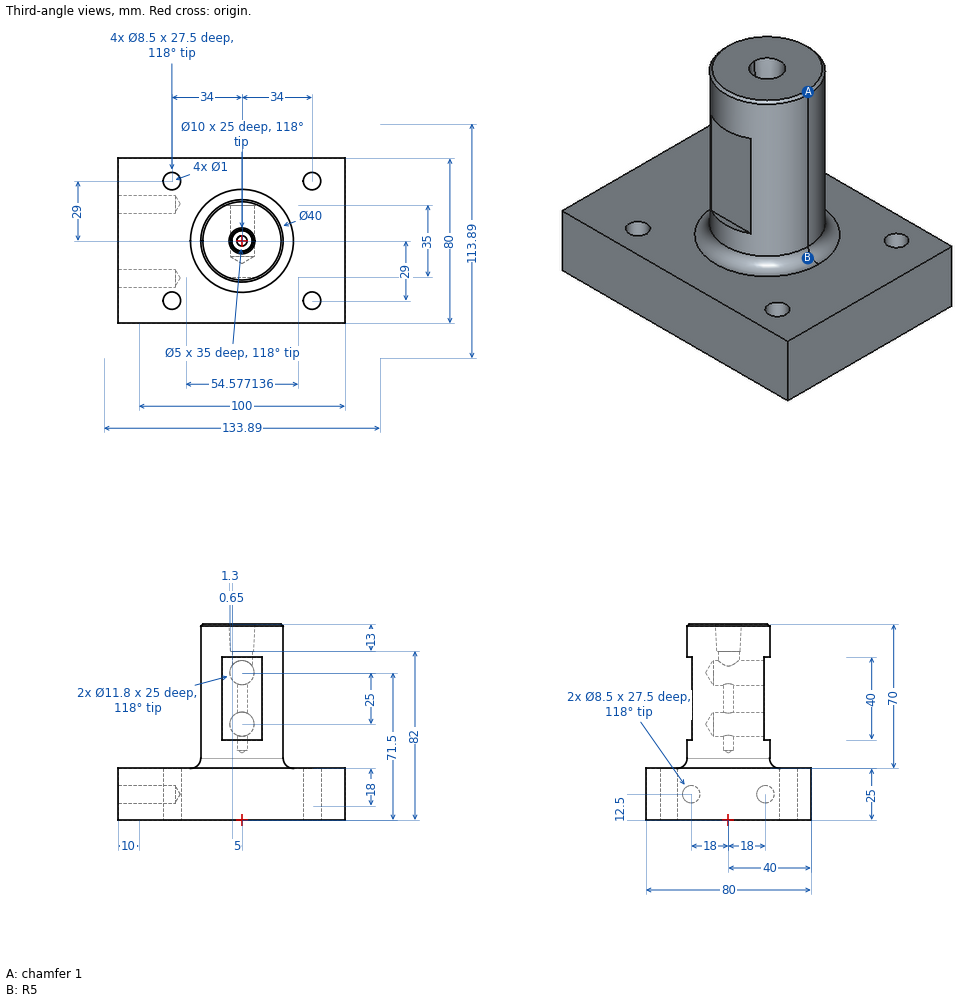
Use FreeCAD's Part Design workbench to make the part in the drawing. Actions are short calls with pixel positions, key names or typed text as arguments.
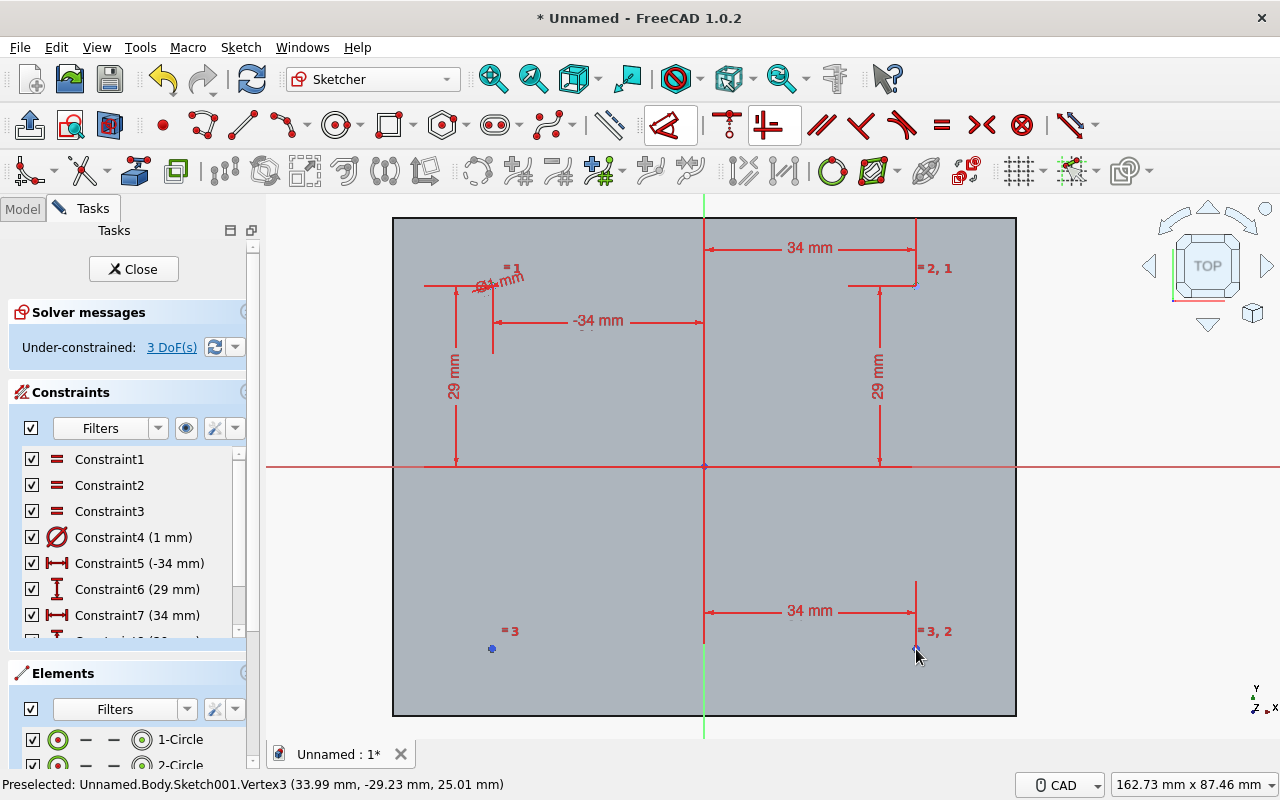
click(916, 649)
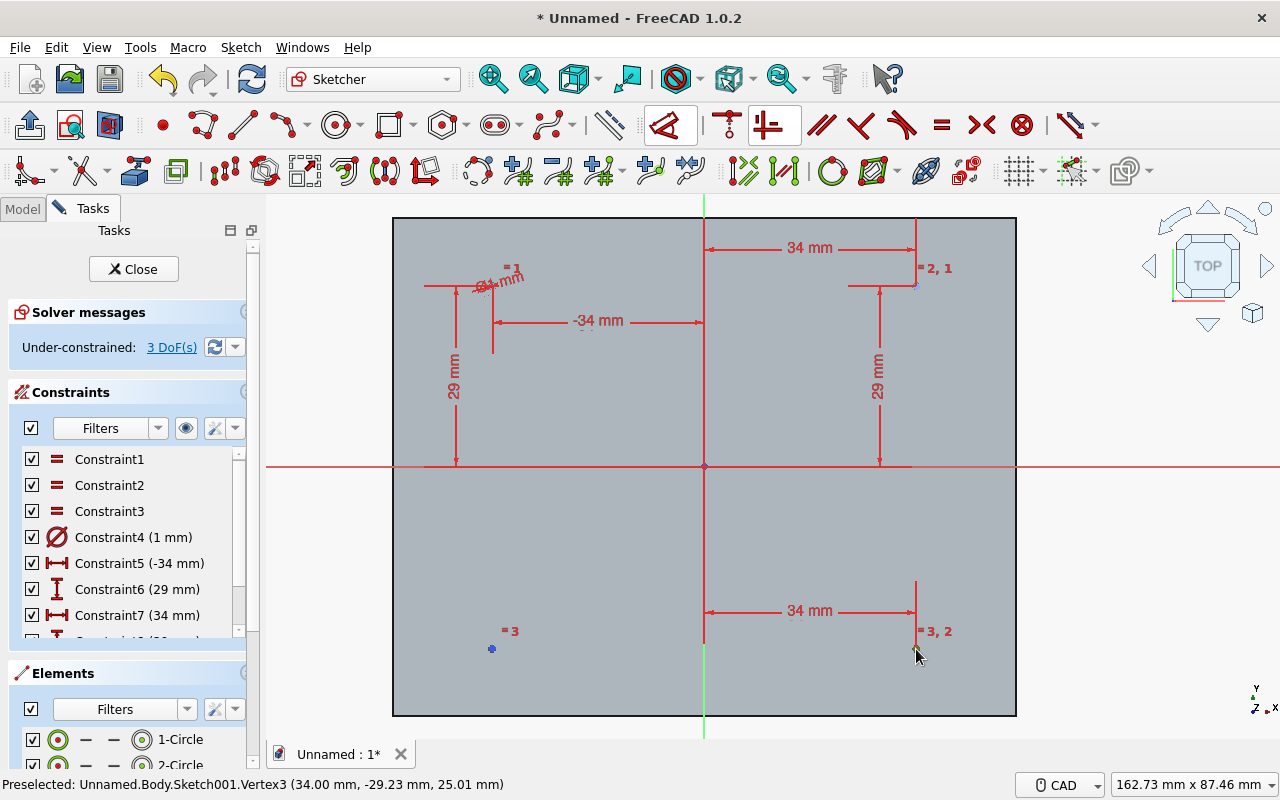
key(i)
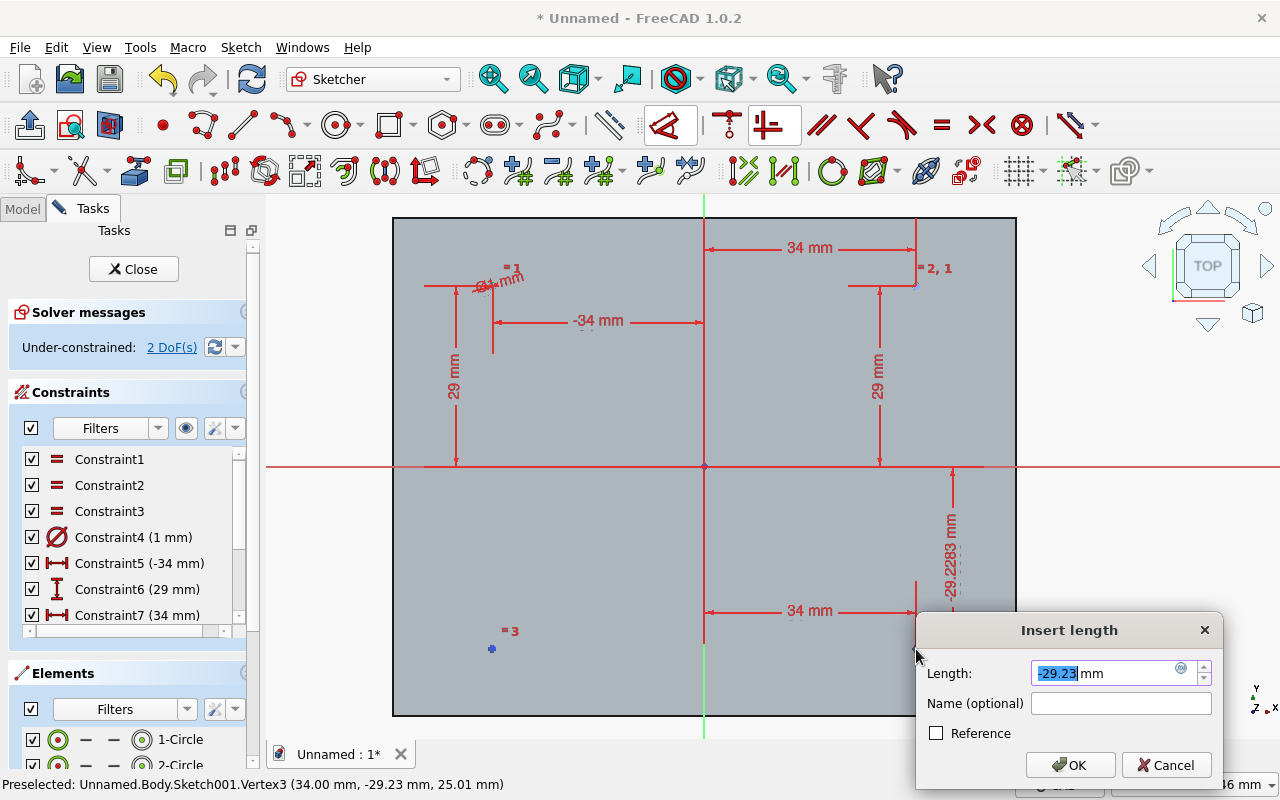
text(-29)
key(Return)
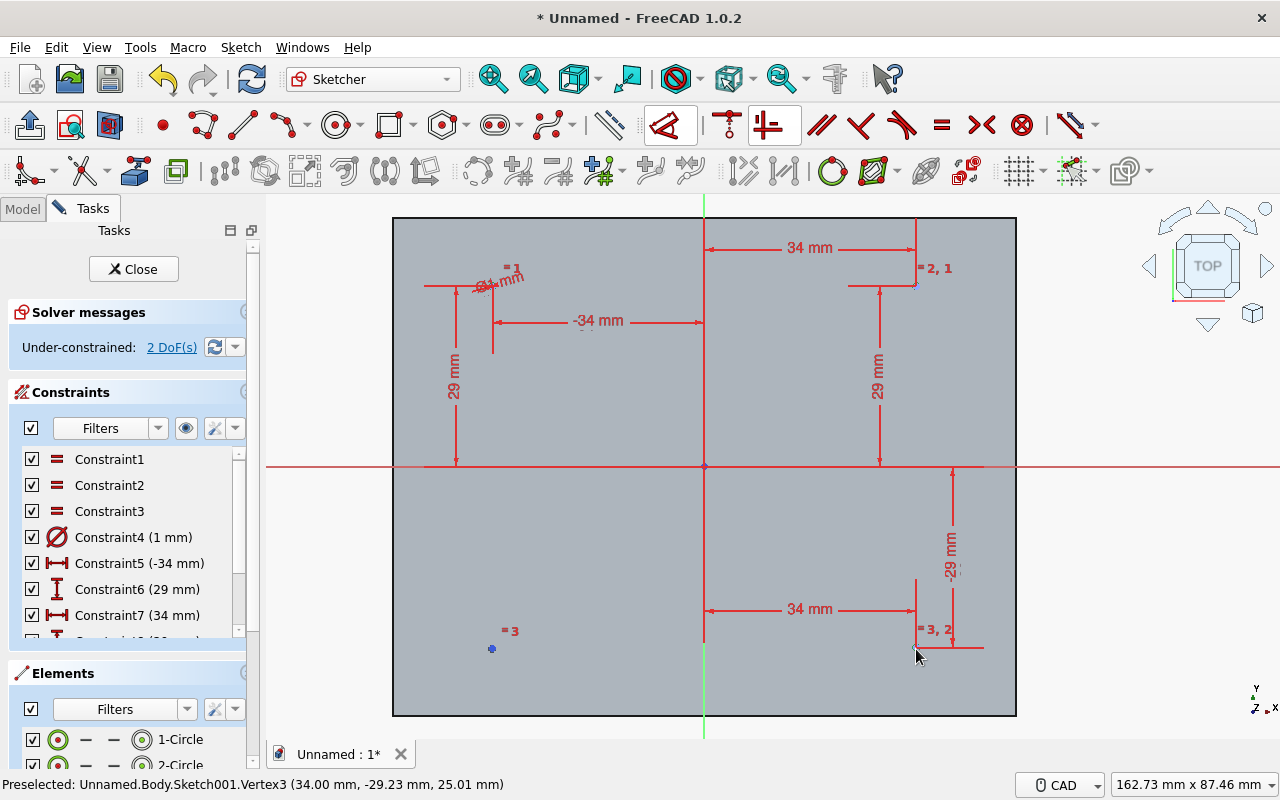
click(492, 649)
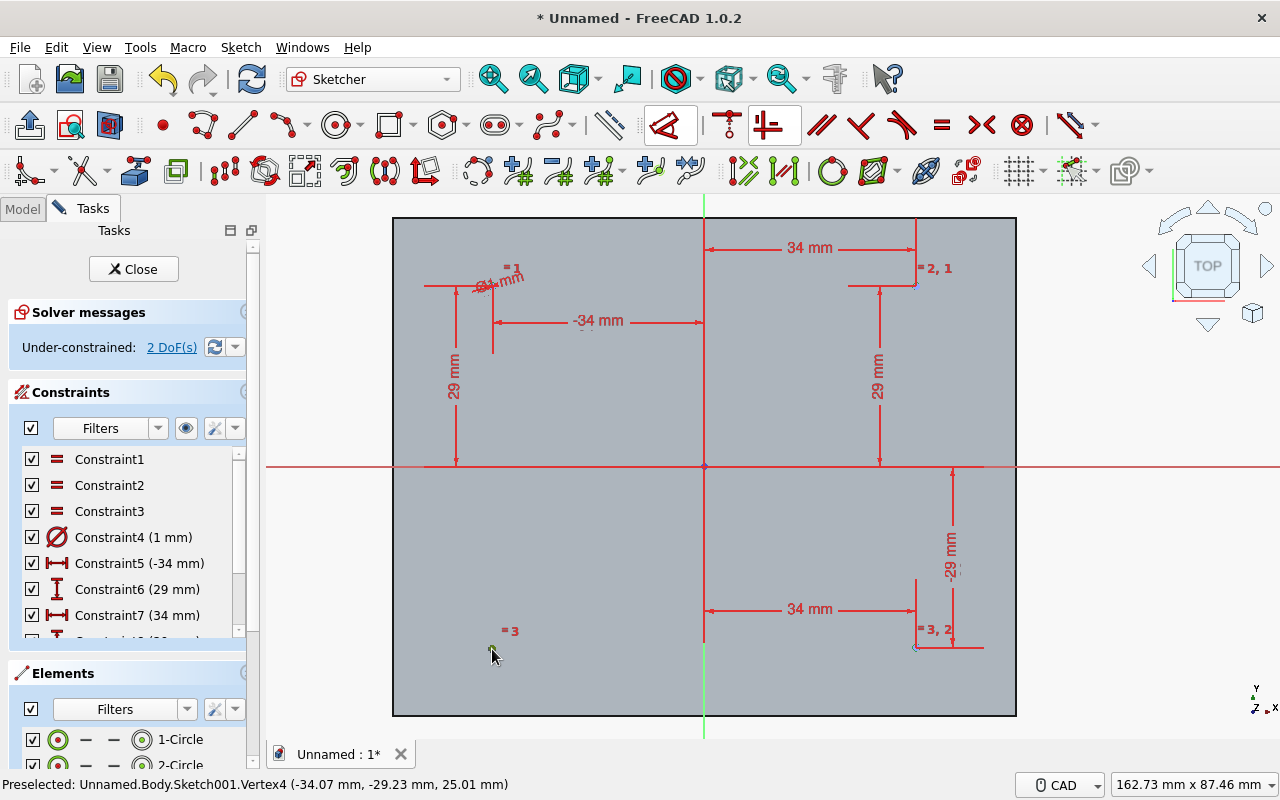
click(692, 126)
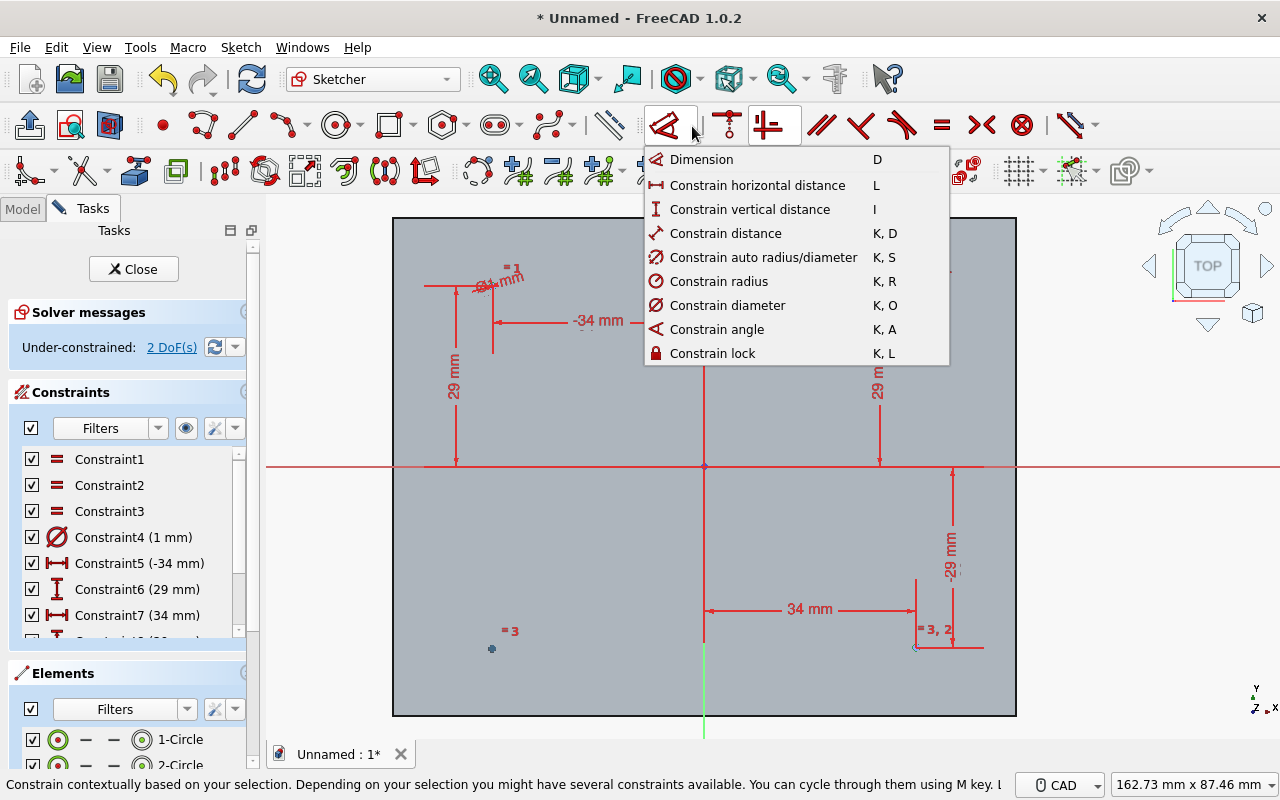
click(797, 185)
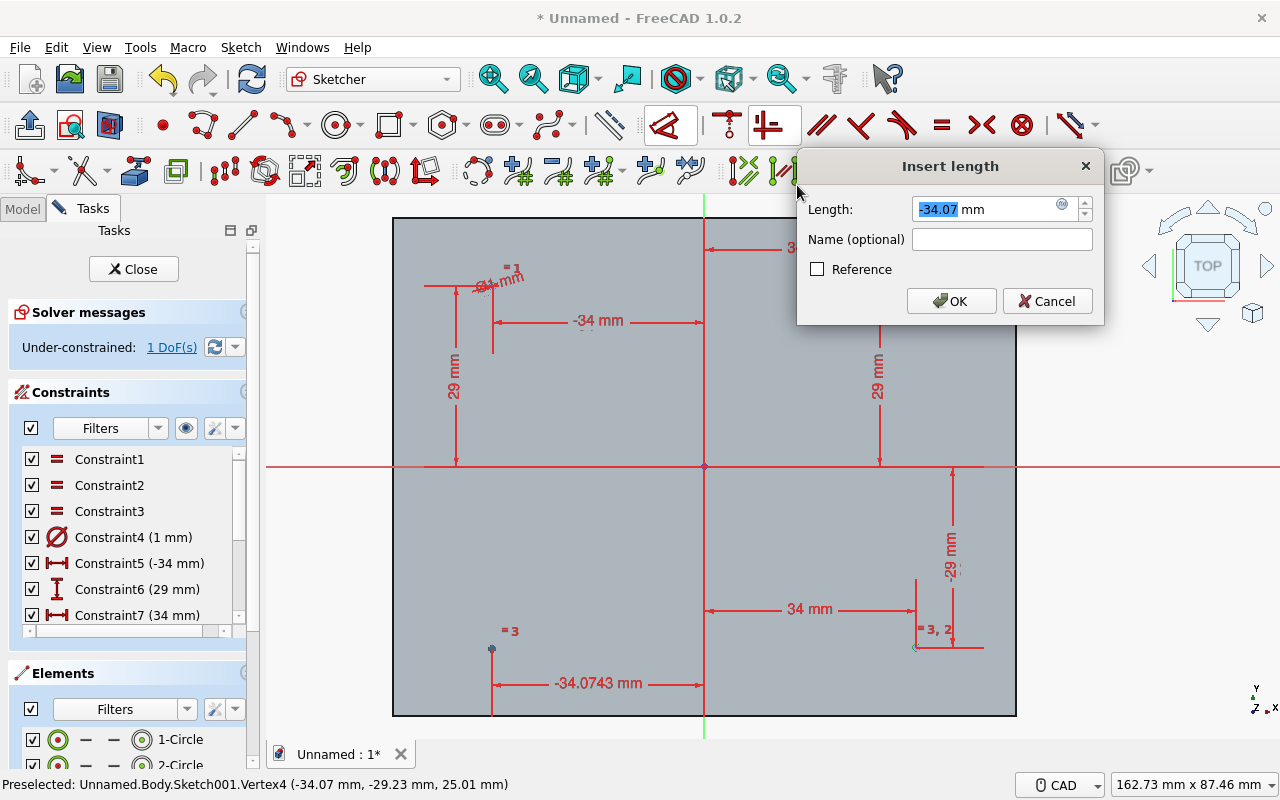
text(-34)
key(Return)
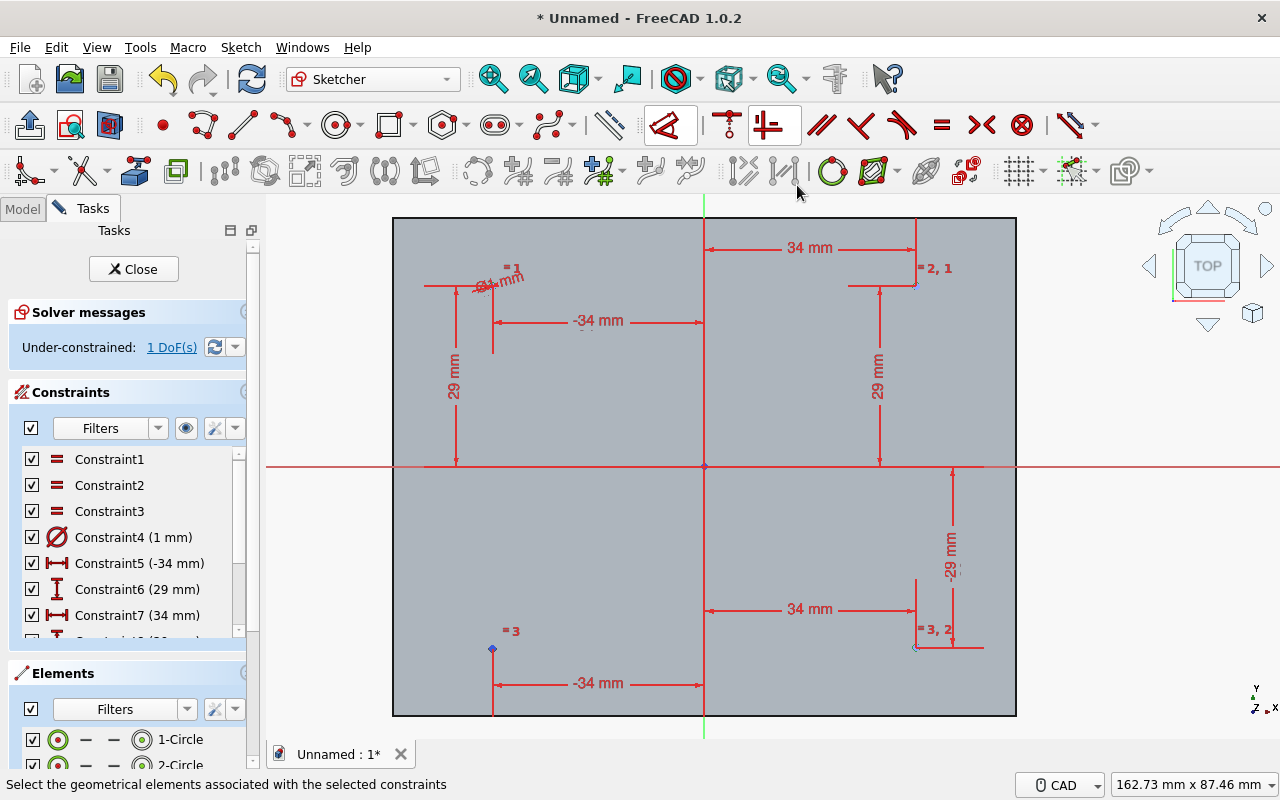
click(493, 649)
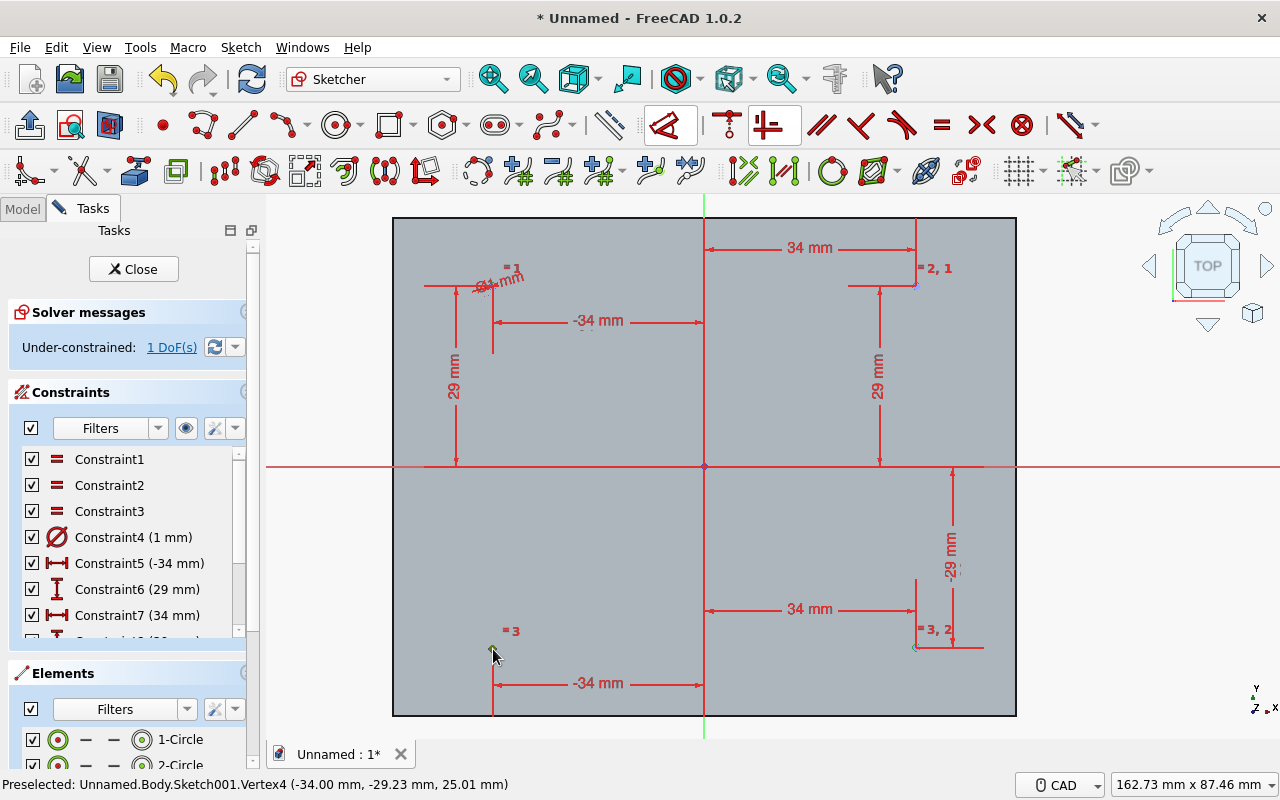
key(i)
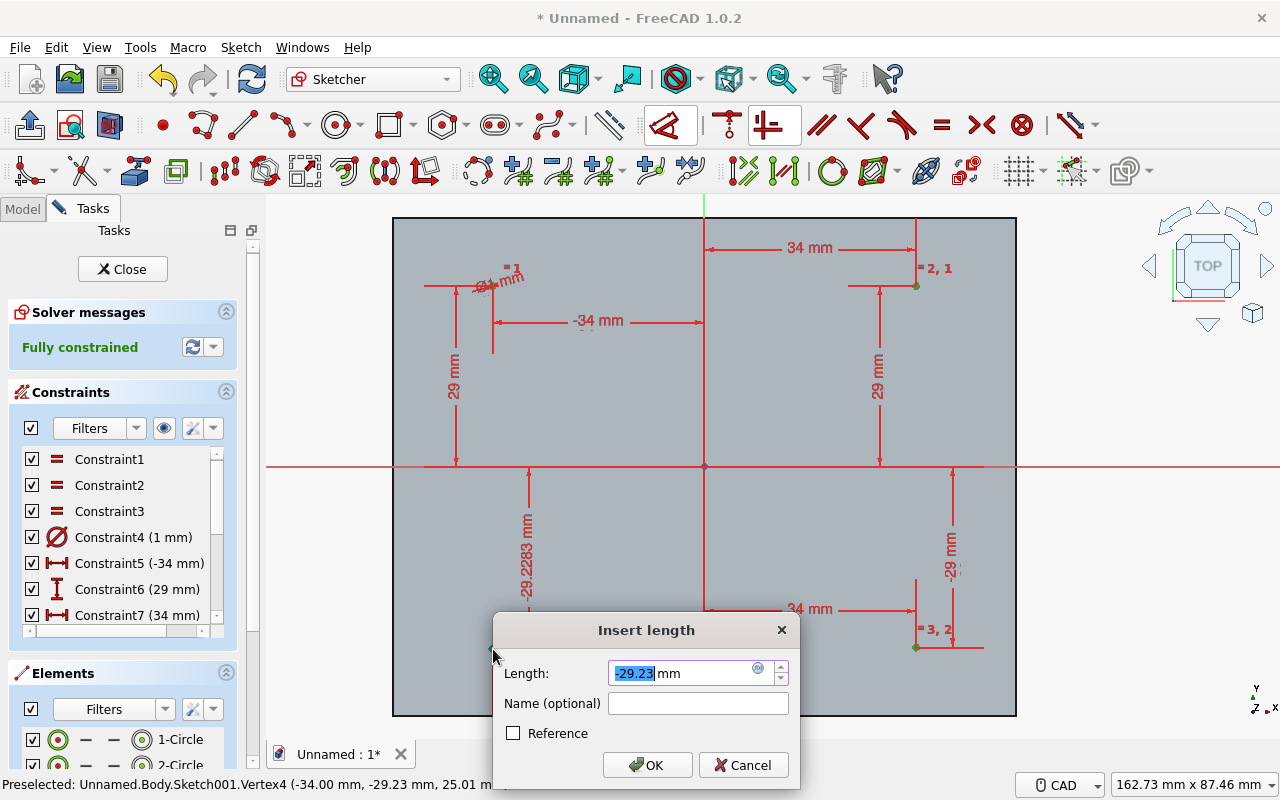
text(-29)
key(Return)